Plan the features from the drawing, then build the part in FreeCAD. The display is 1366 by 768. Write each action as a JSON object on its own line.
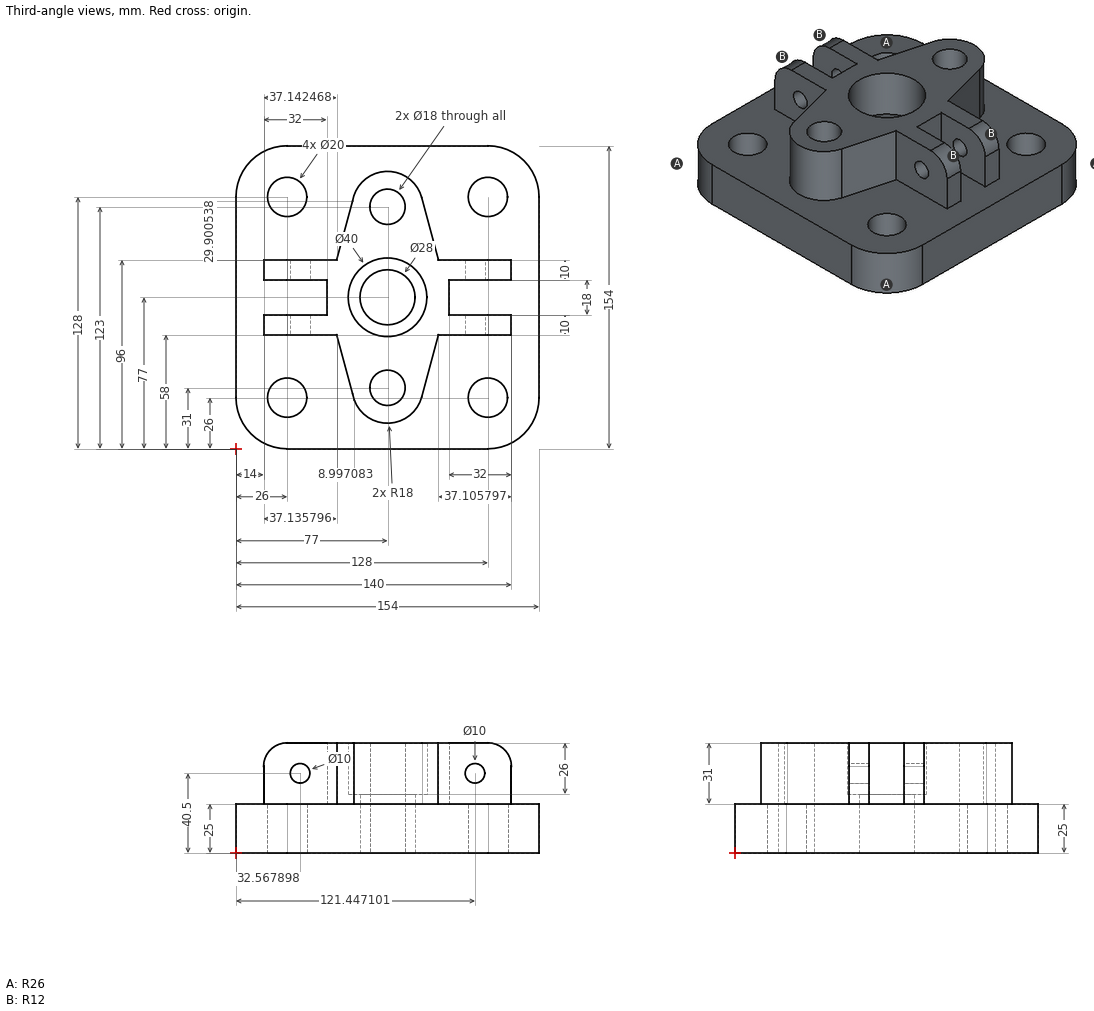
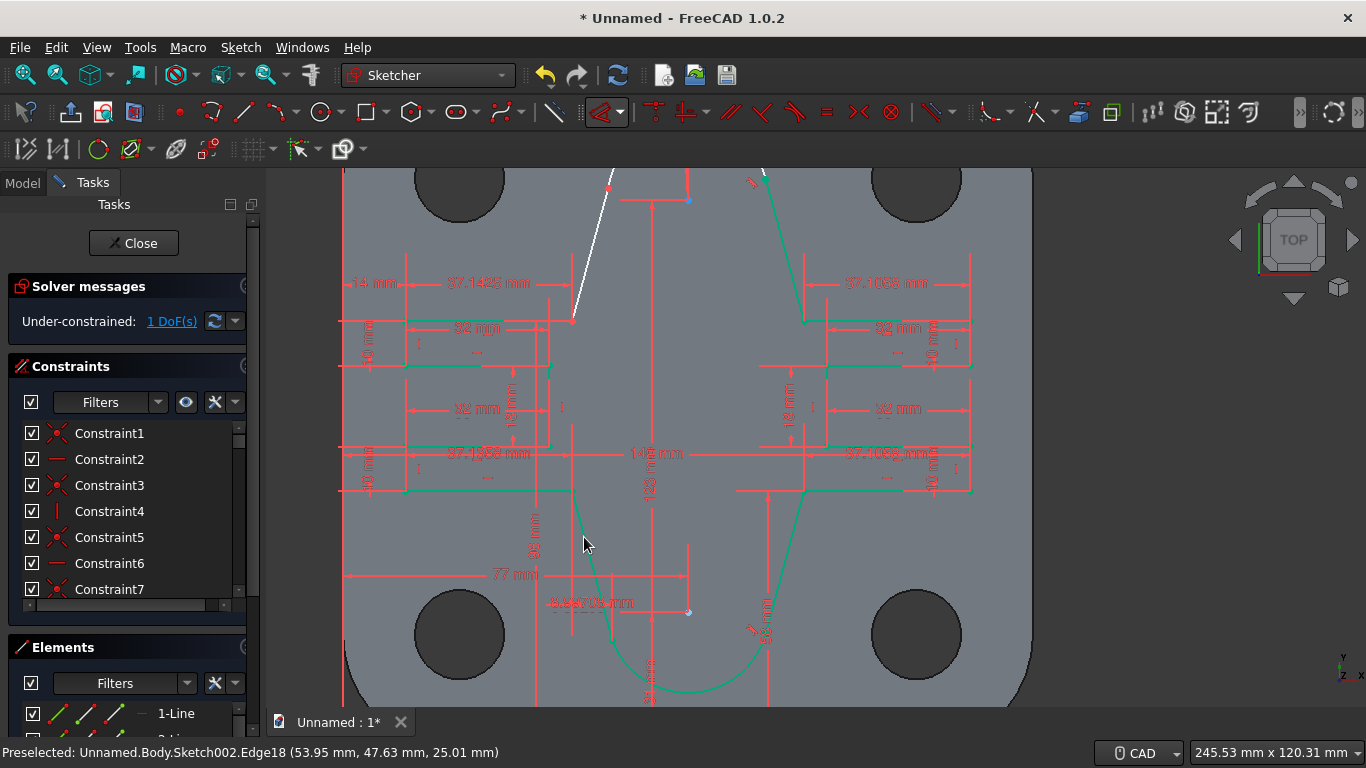
{"action": "left_click", "coordinate": [597, 228]}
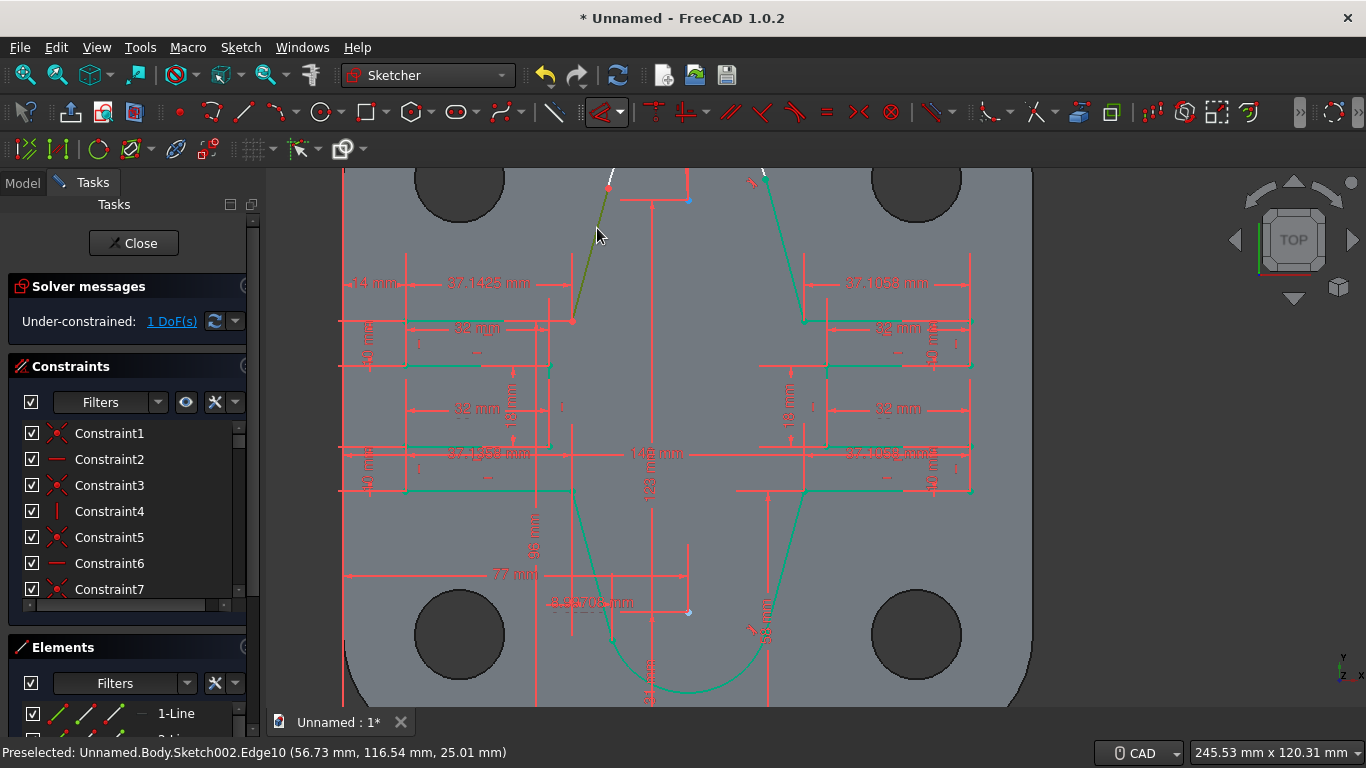
{"action": "left_click", "coordinate": [622, 112]}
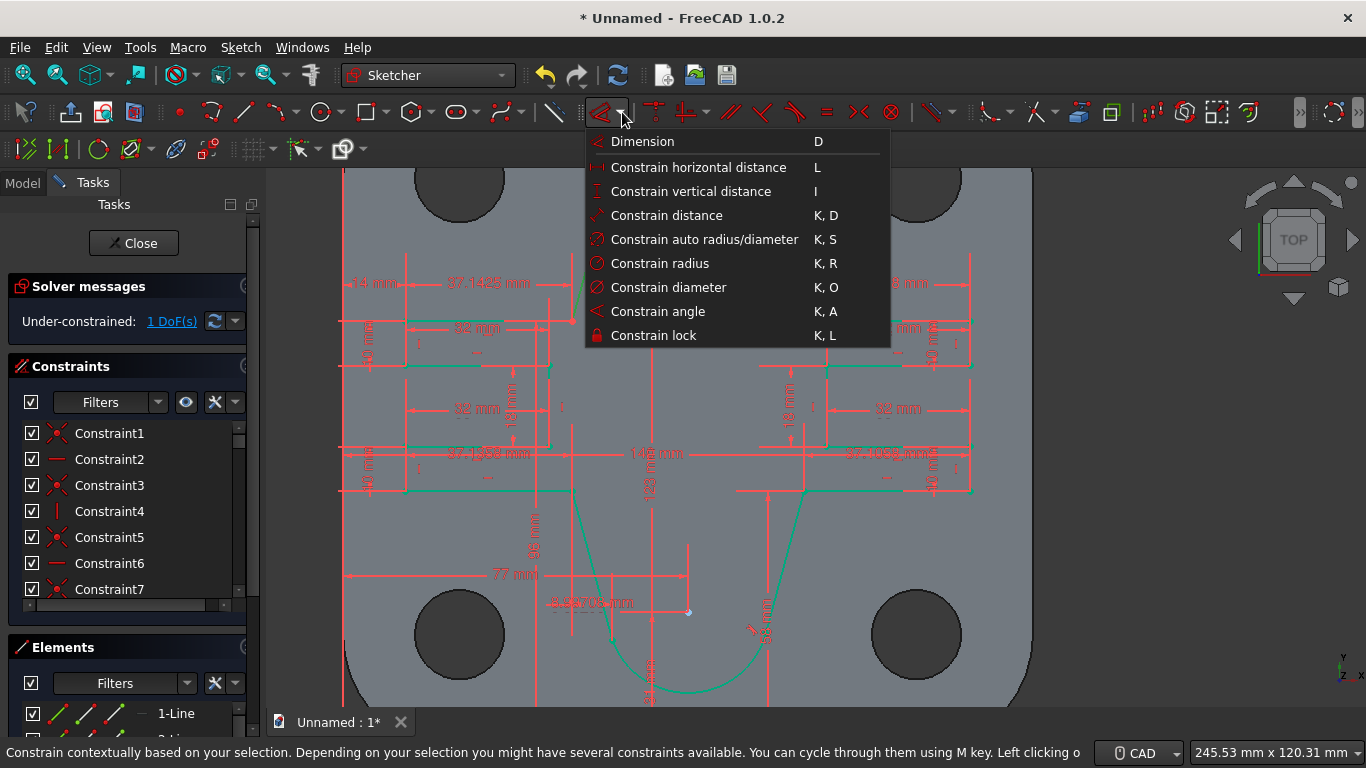
{"action": "left_click", "coordinate": [738, 191]}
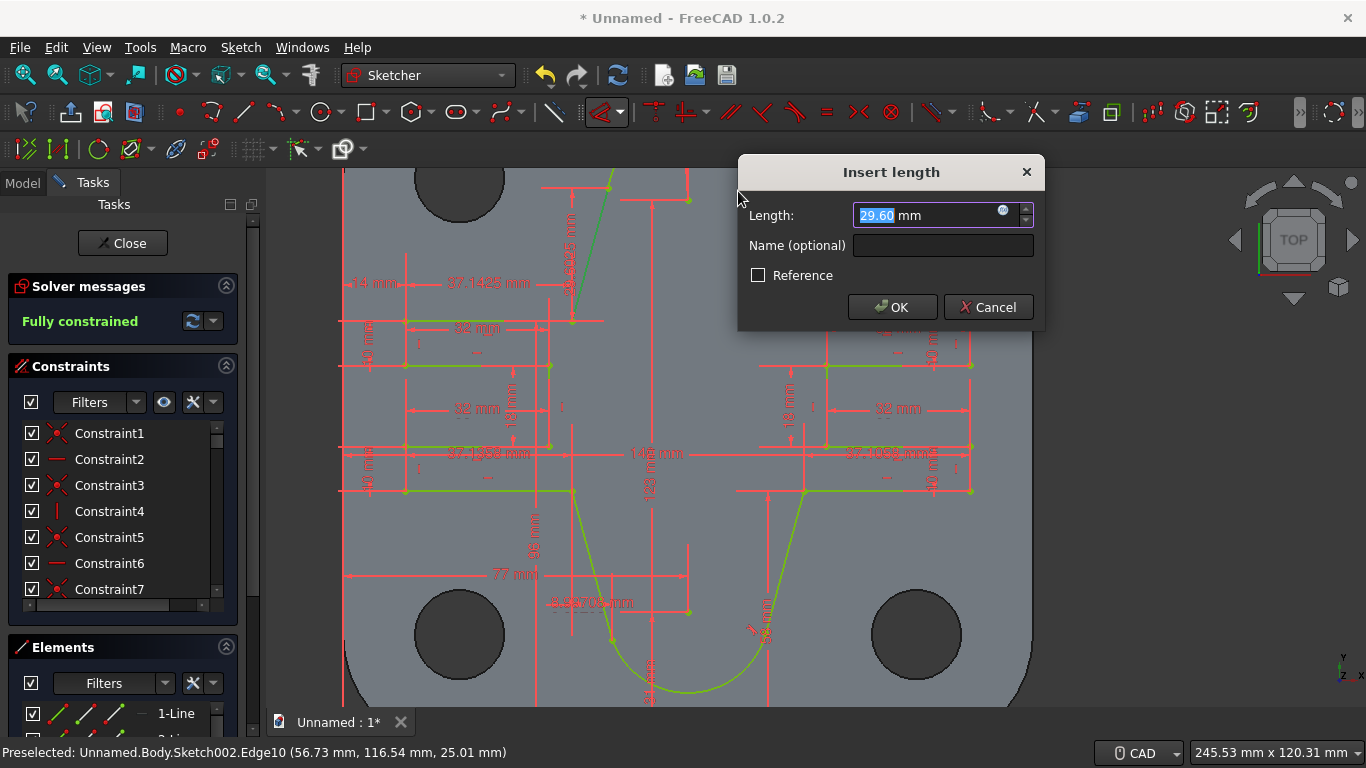
{"action": "type", "text": "29.900538"}
{"action": "key", "text": "Return"}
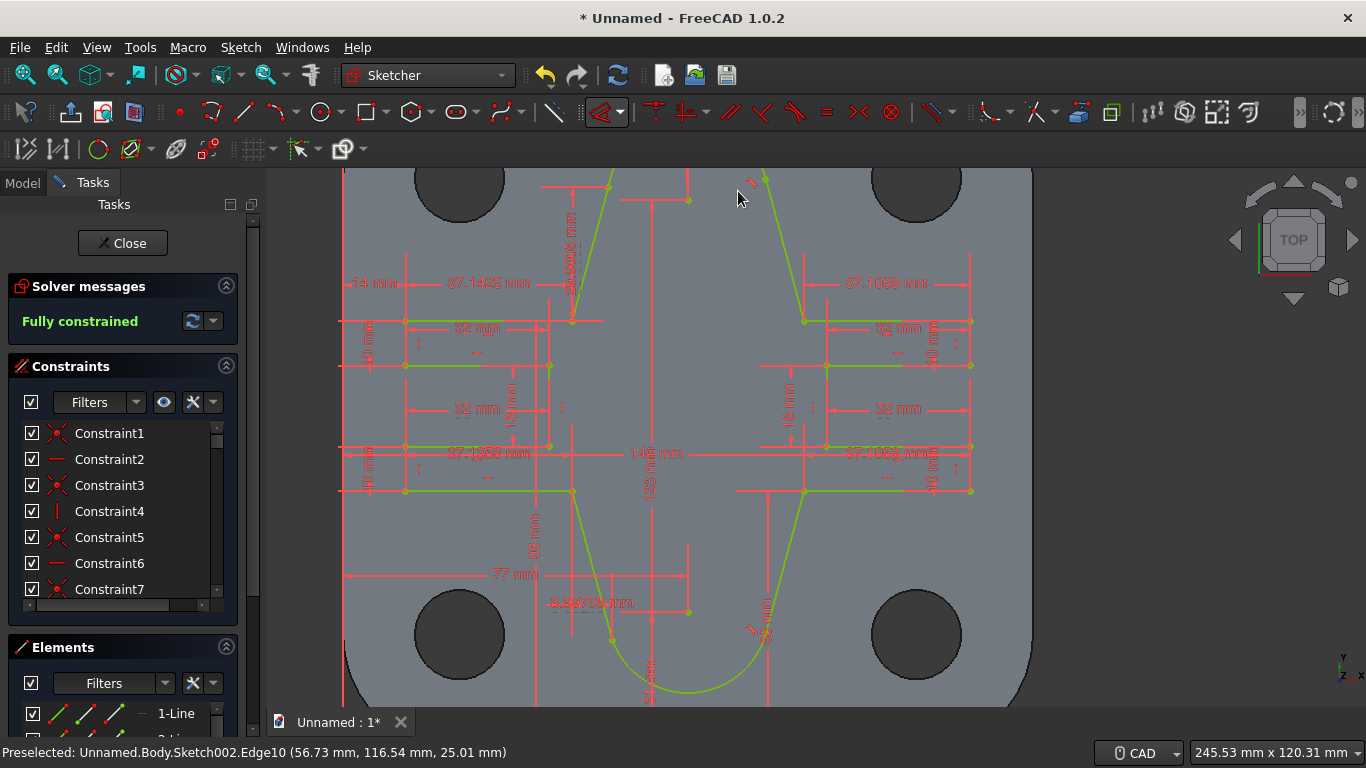
{"action": "left_click", "coordinate": [123, 243]}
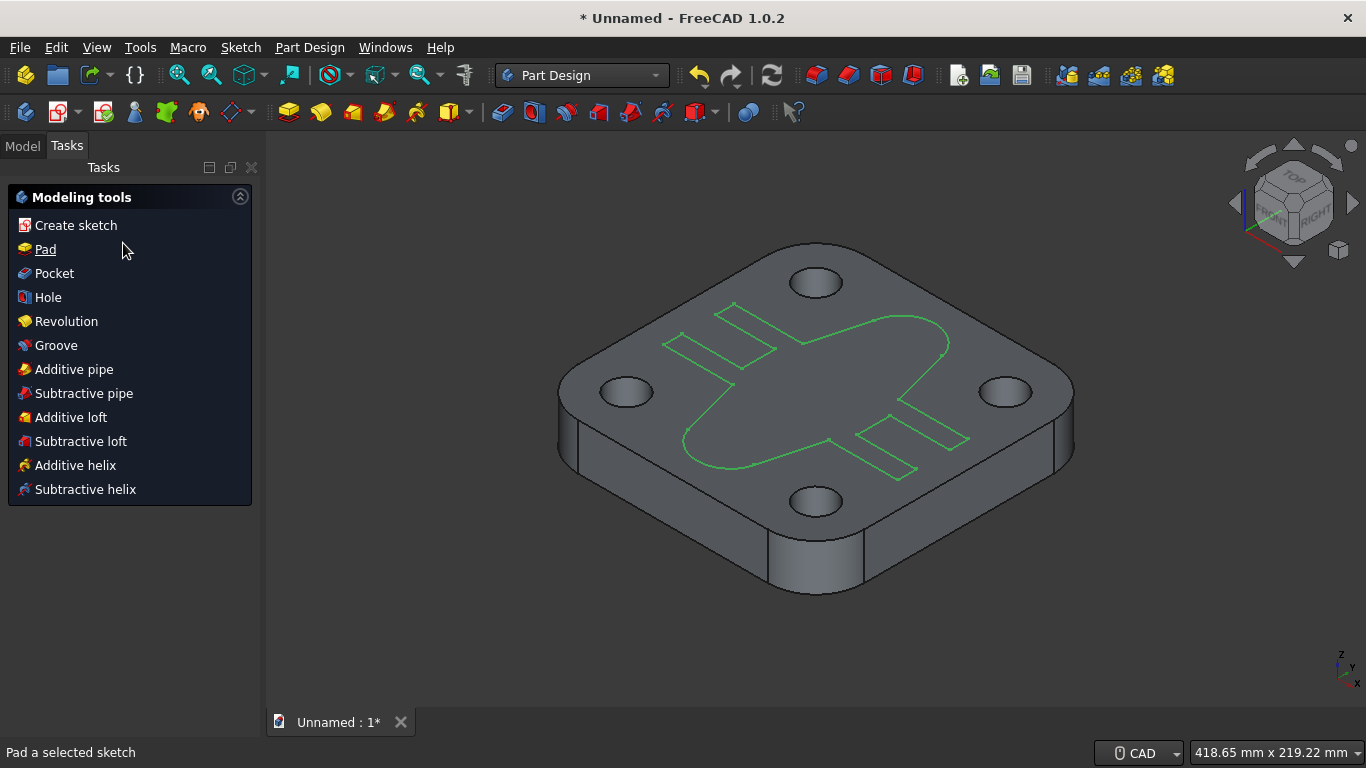
{"action": "left_click", "coordinate": [290, 112]}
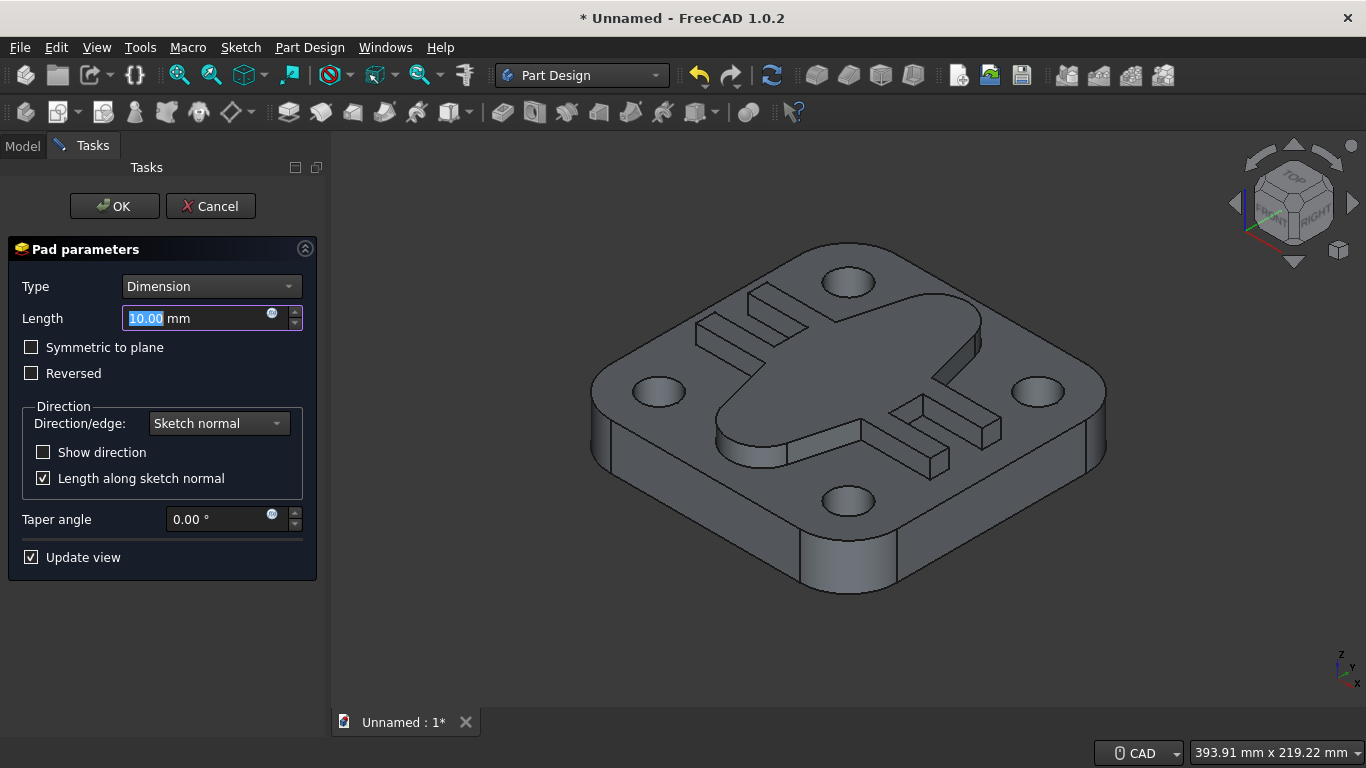
{"action": "type", "text": "31"}
{"action": "key", "text": "Tab"}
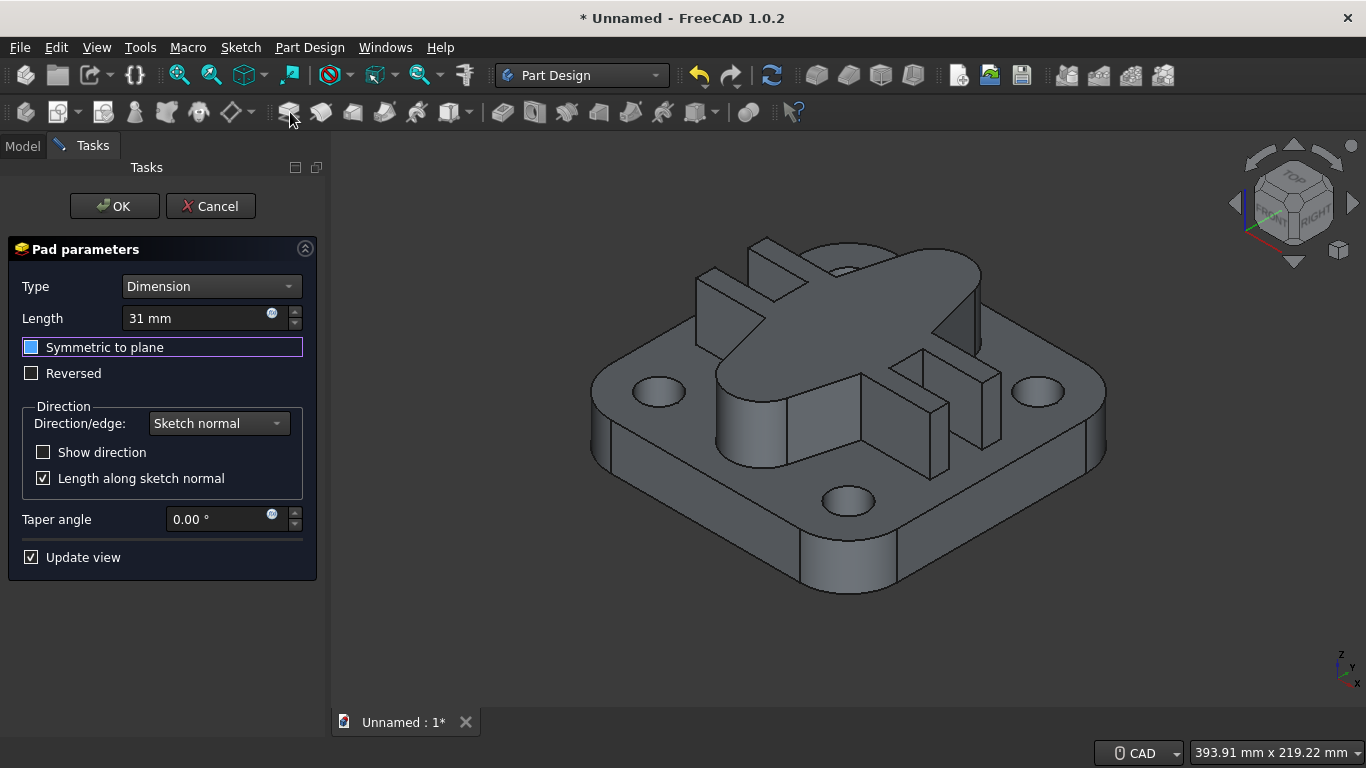
{"action": "left_click", "coordinate": [115, 206]}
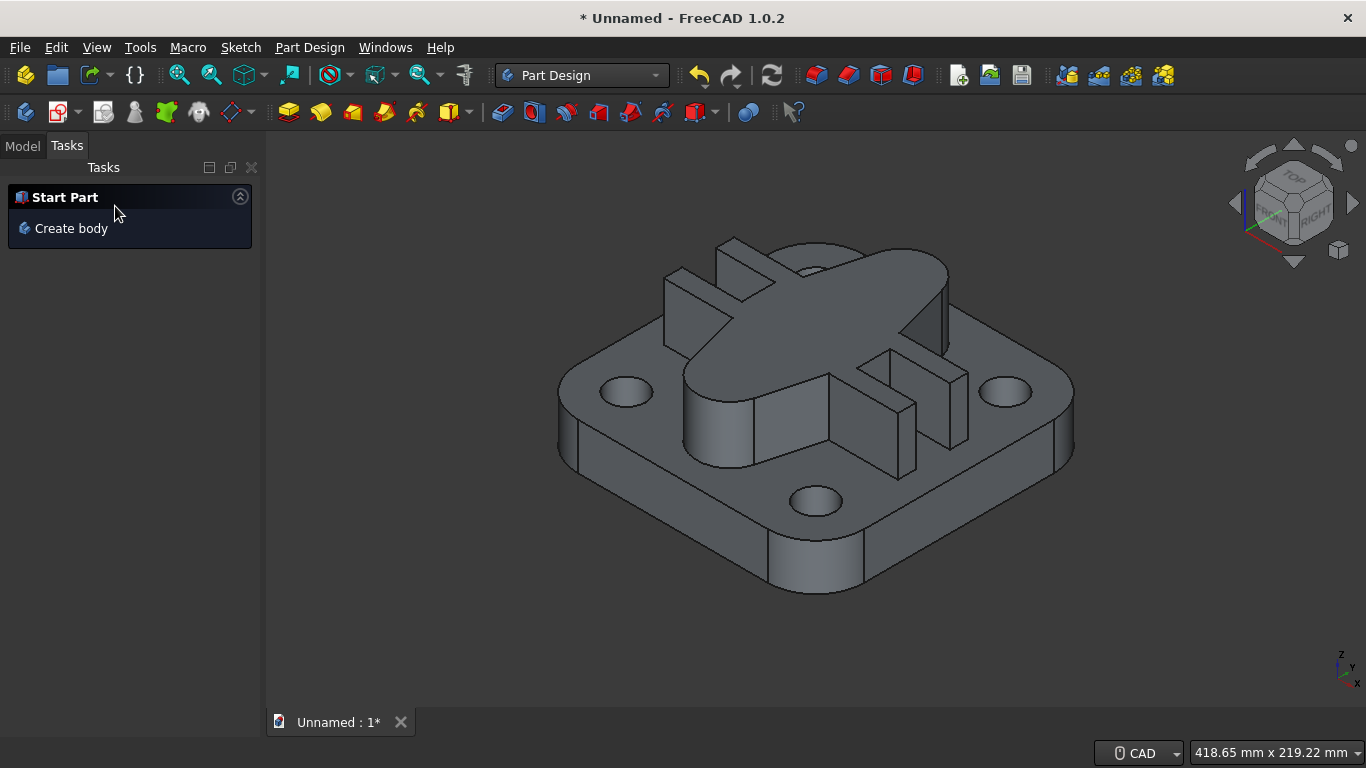
{"action": "left_click", "coordinate": [816, 324]}